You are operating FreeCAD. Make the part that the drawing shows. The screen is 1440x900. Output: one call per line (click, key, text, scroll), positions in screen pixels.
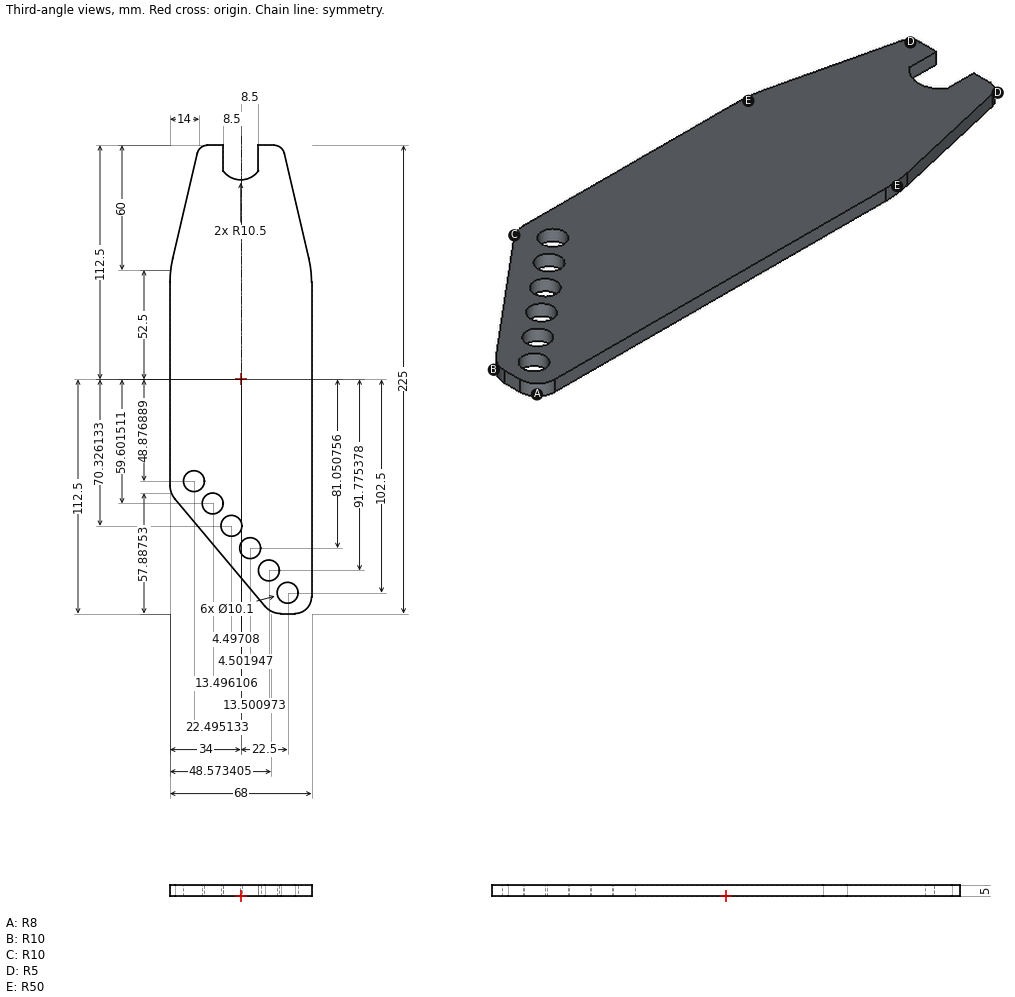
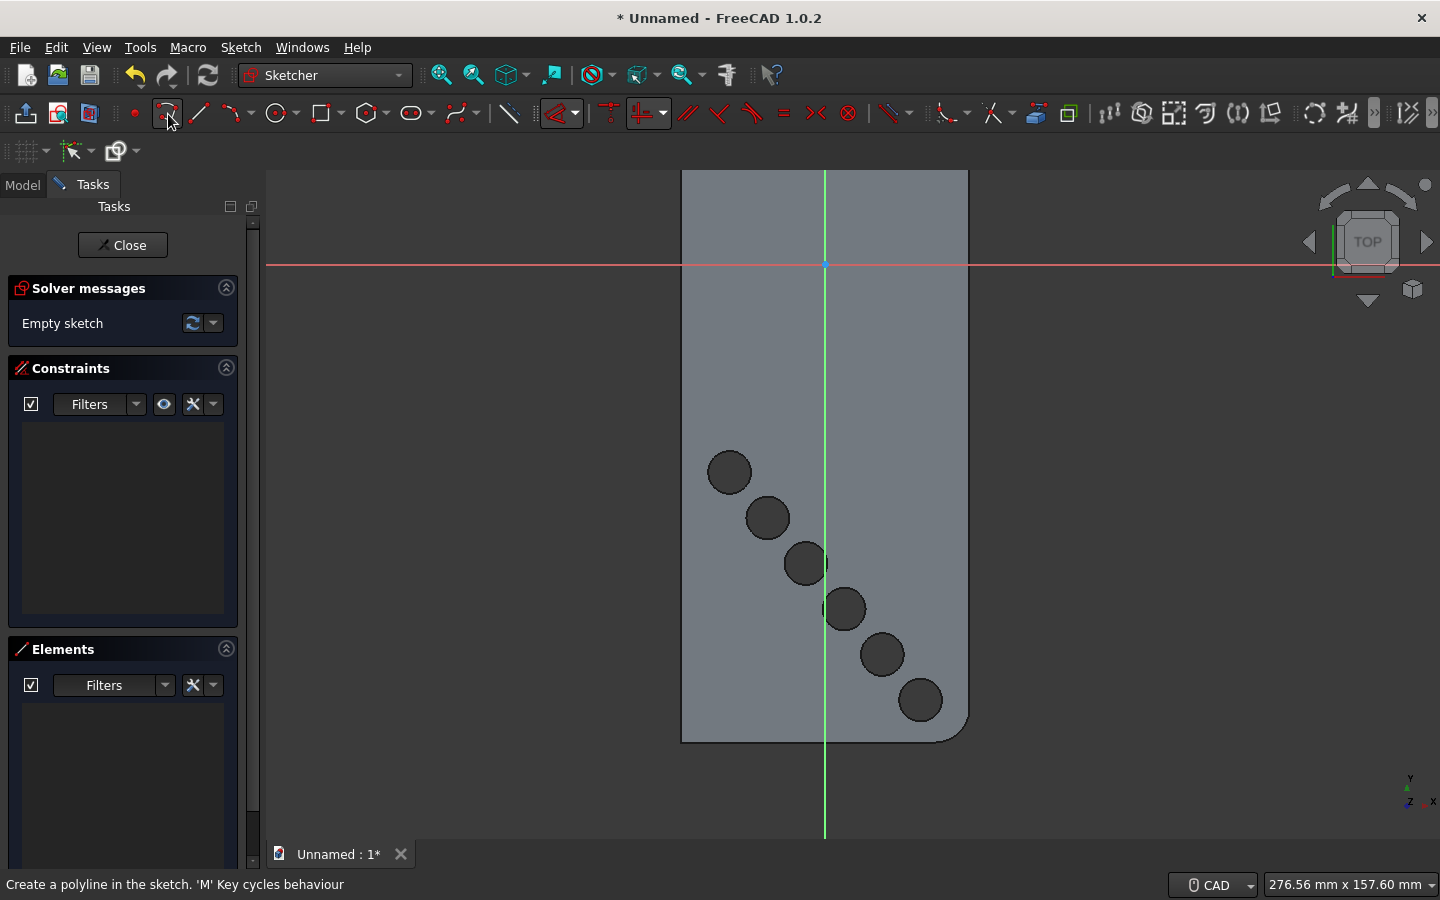
click(681, 497)
click(681, 743)
click(887, 743)
click(681, 498)
key(Escape)
key(Escape)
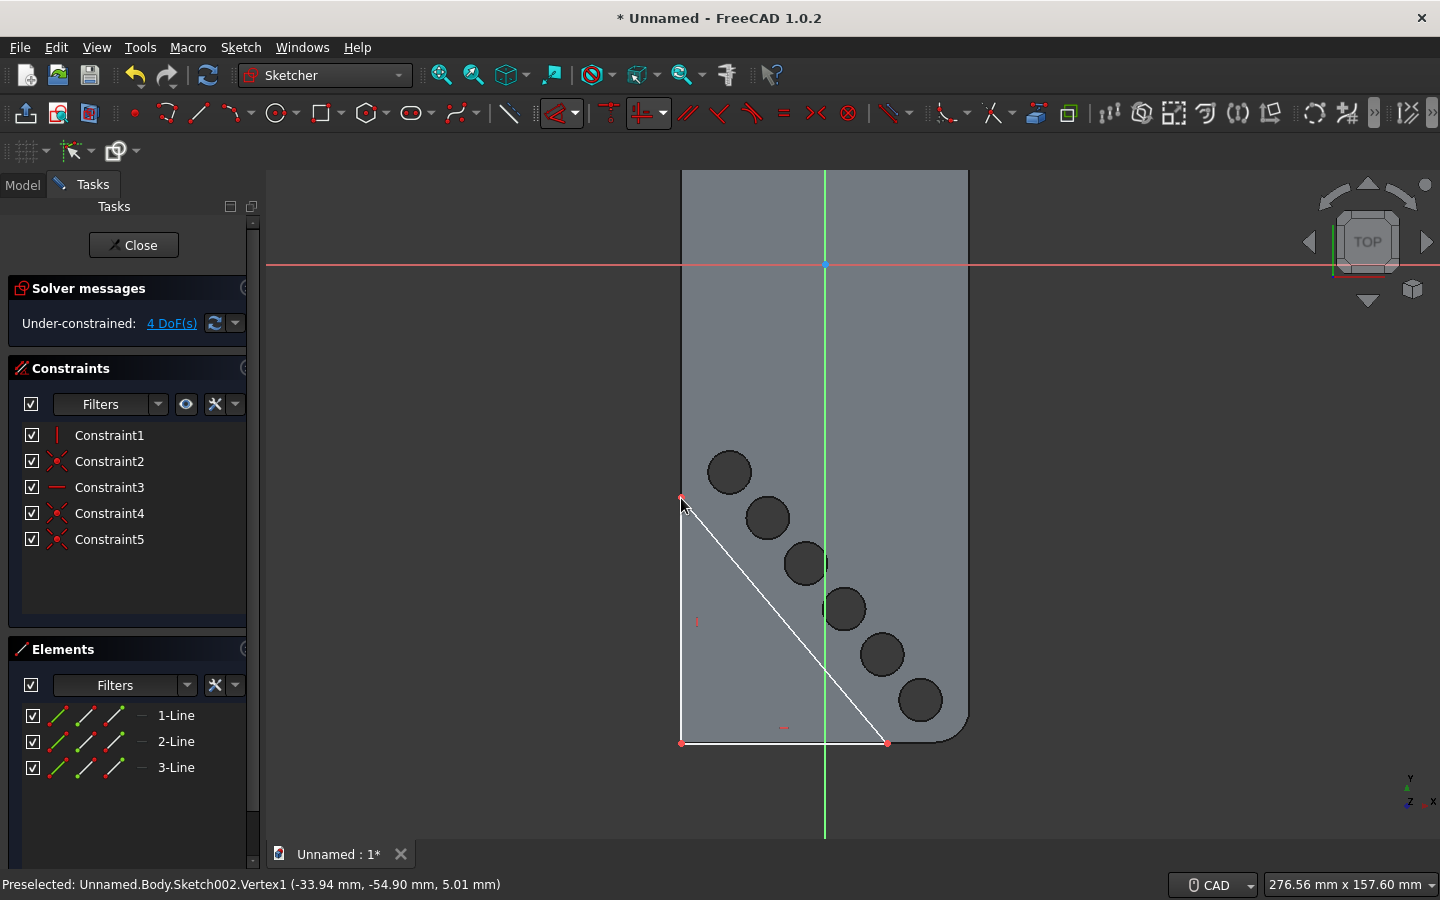
click(681, 498)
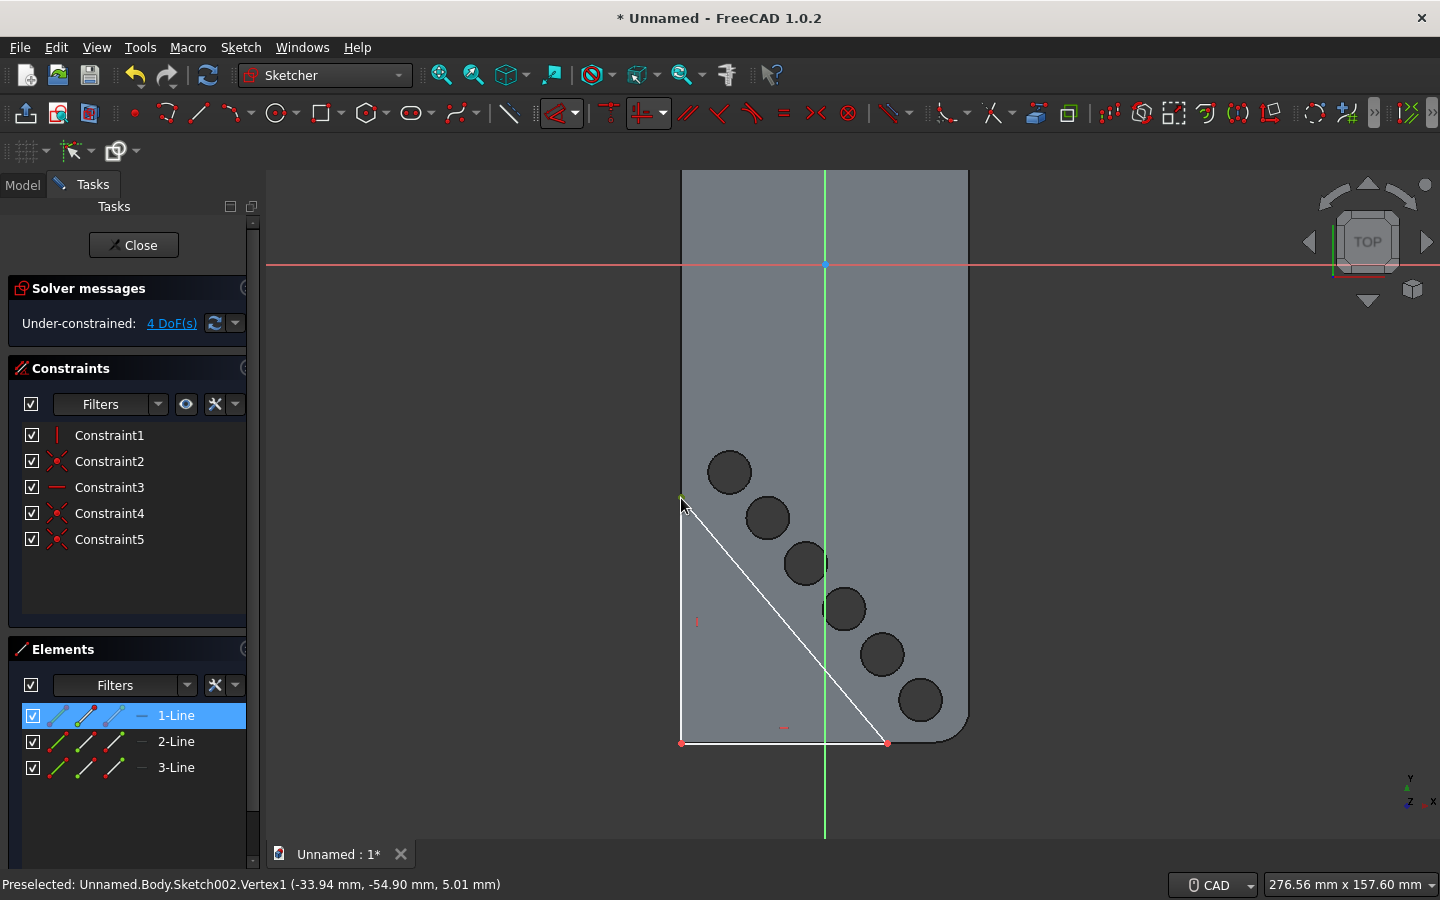
key(l)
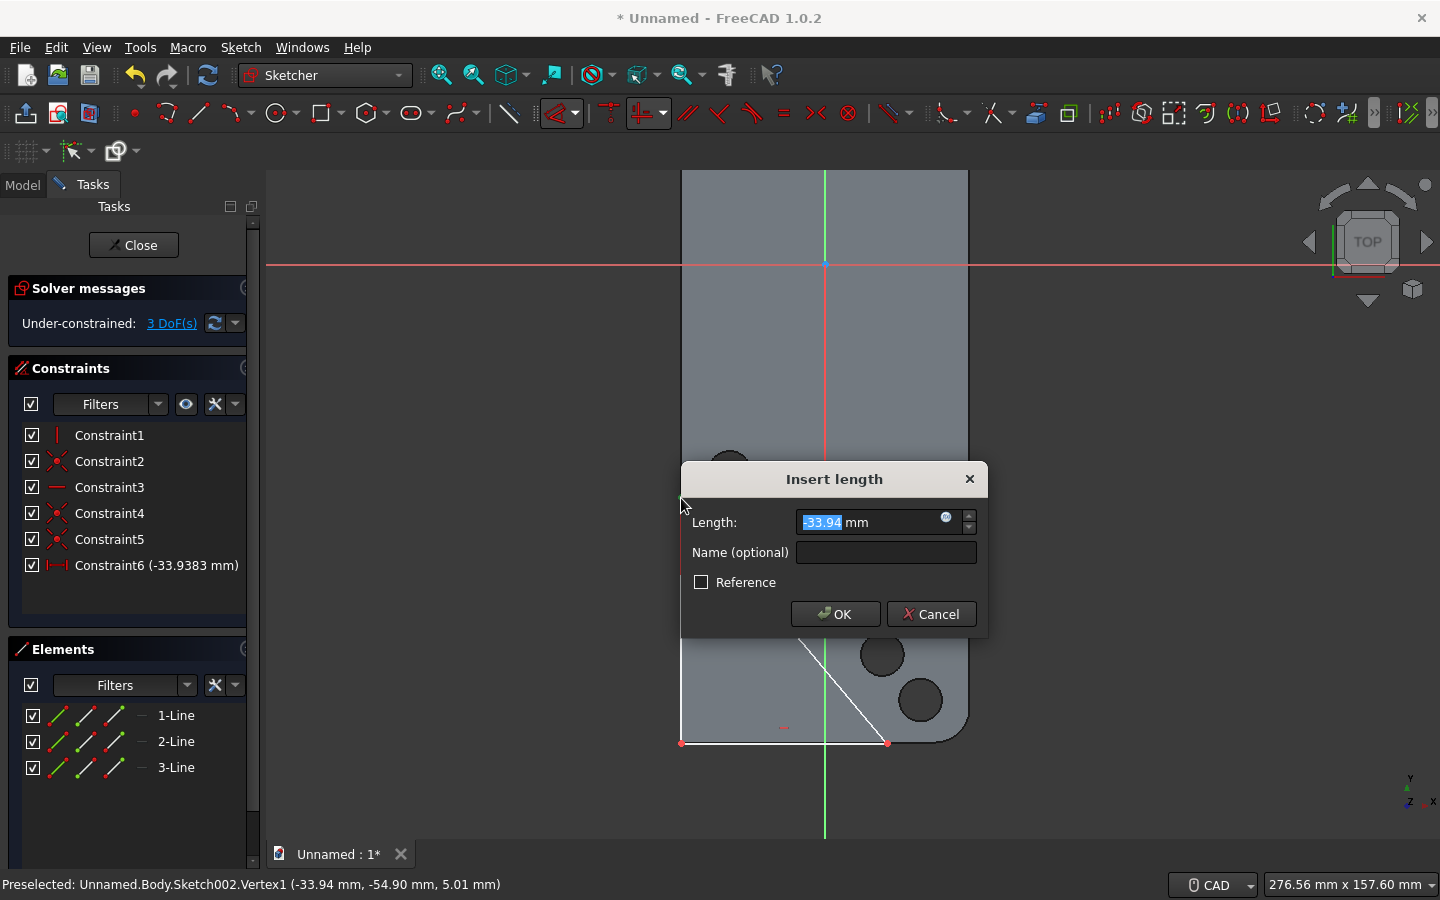
text(-34)
key(Return)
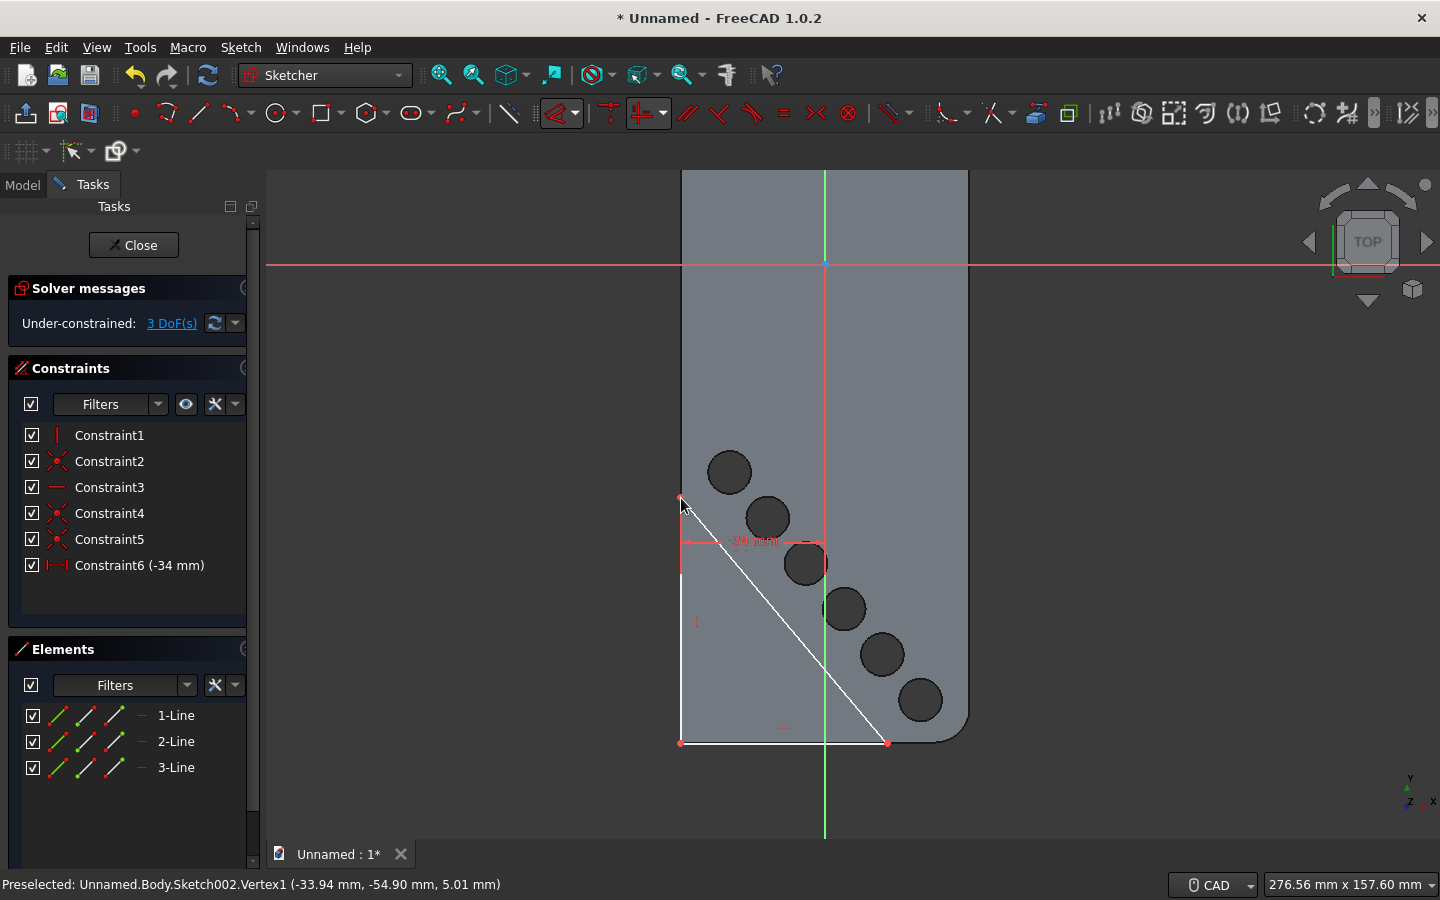
click(681, 744)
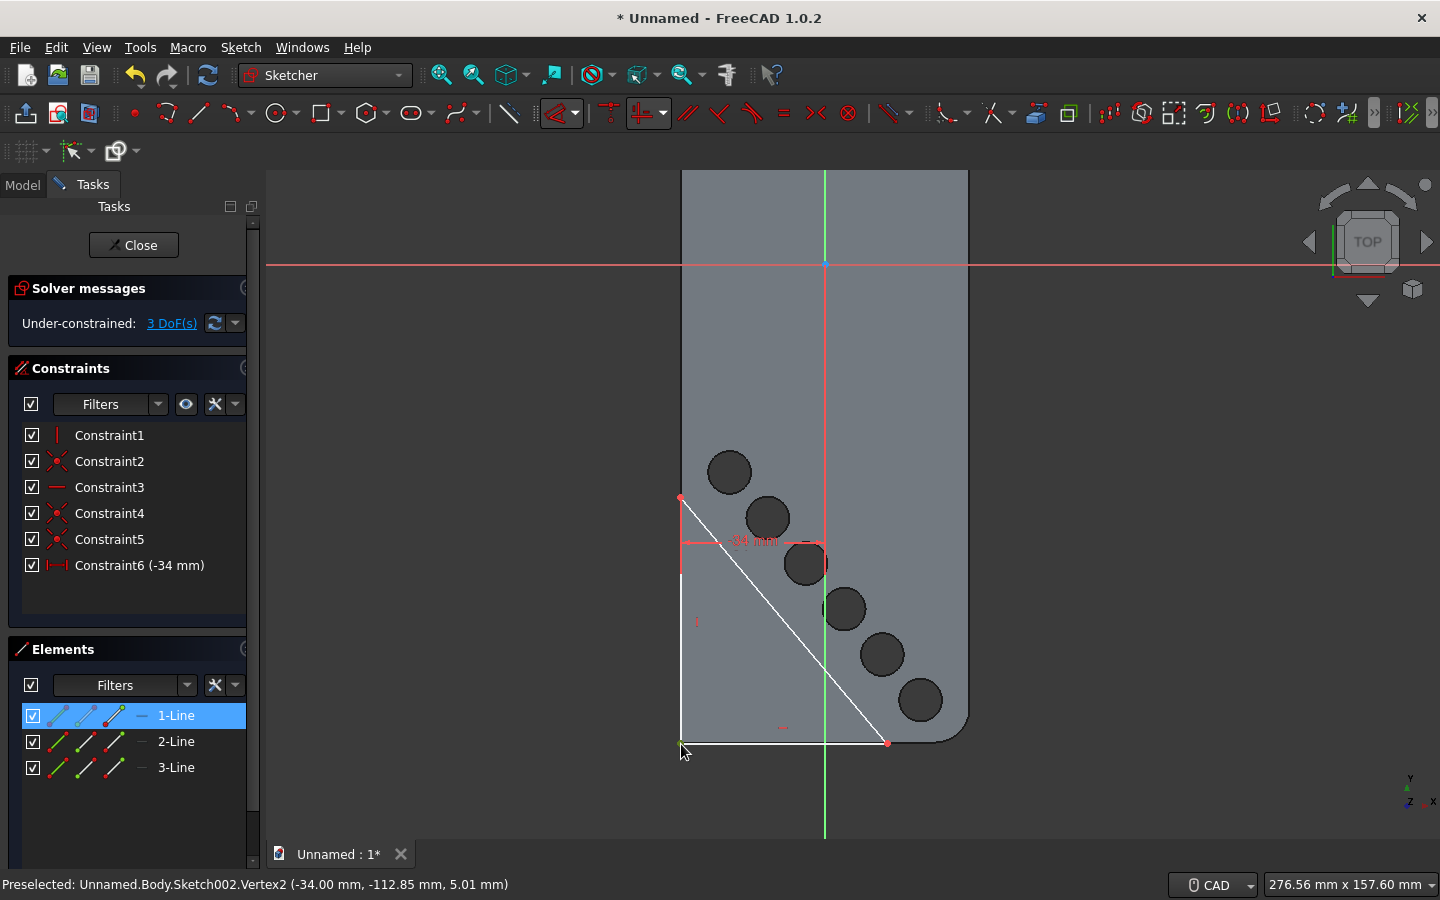
key(i)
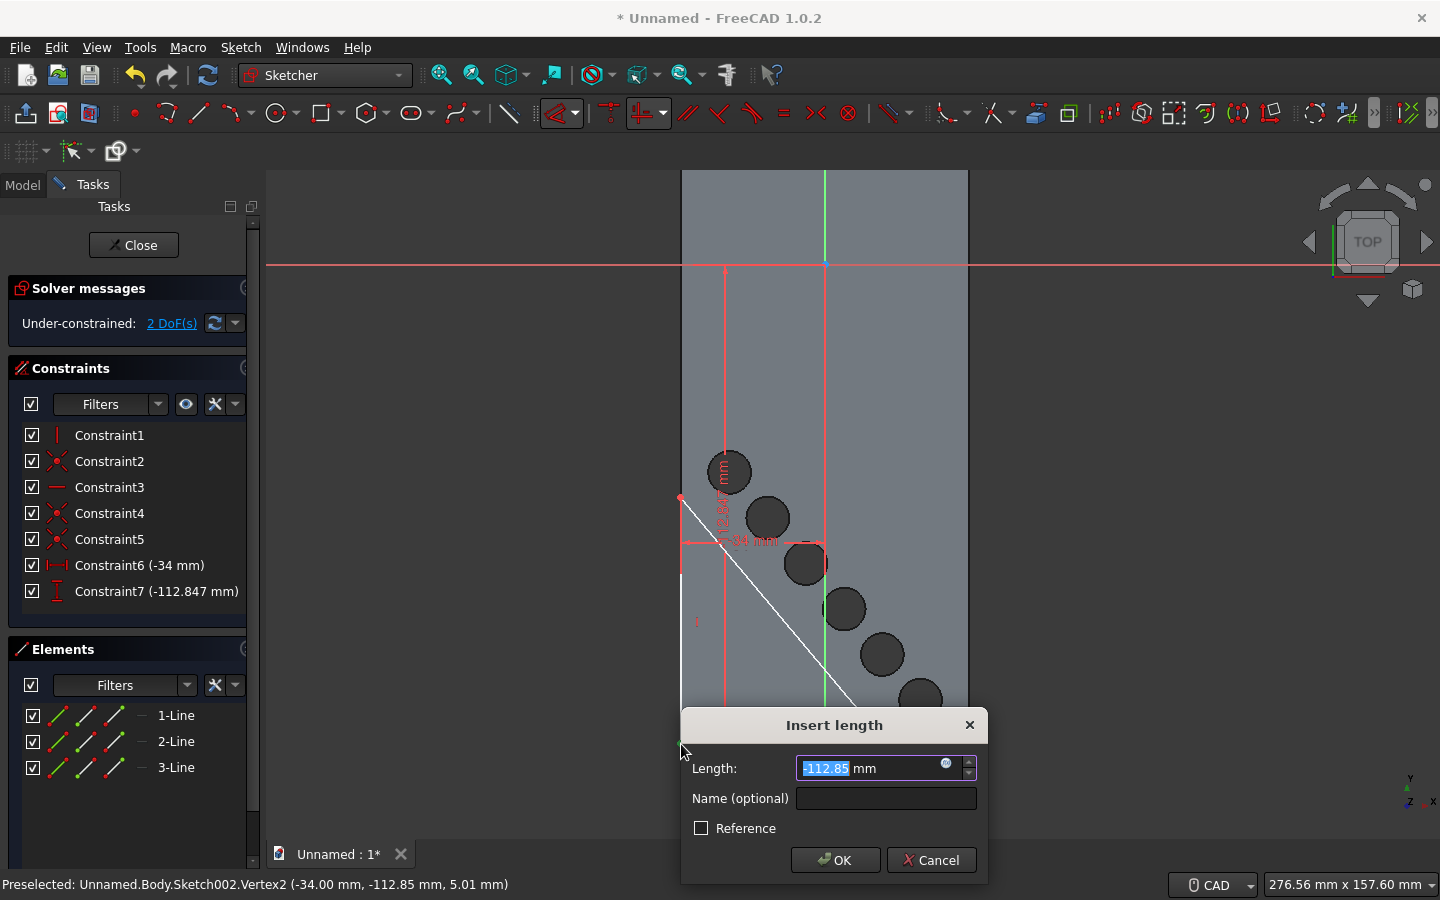
text(-112.5)
key(Return)